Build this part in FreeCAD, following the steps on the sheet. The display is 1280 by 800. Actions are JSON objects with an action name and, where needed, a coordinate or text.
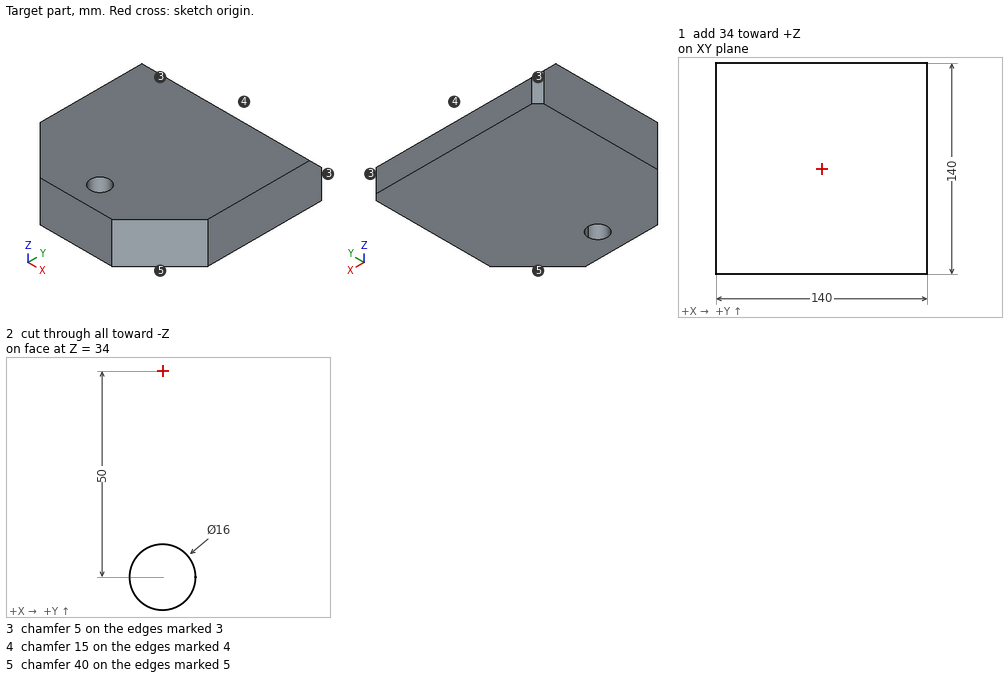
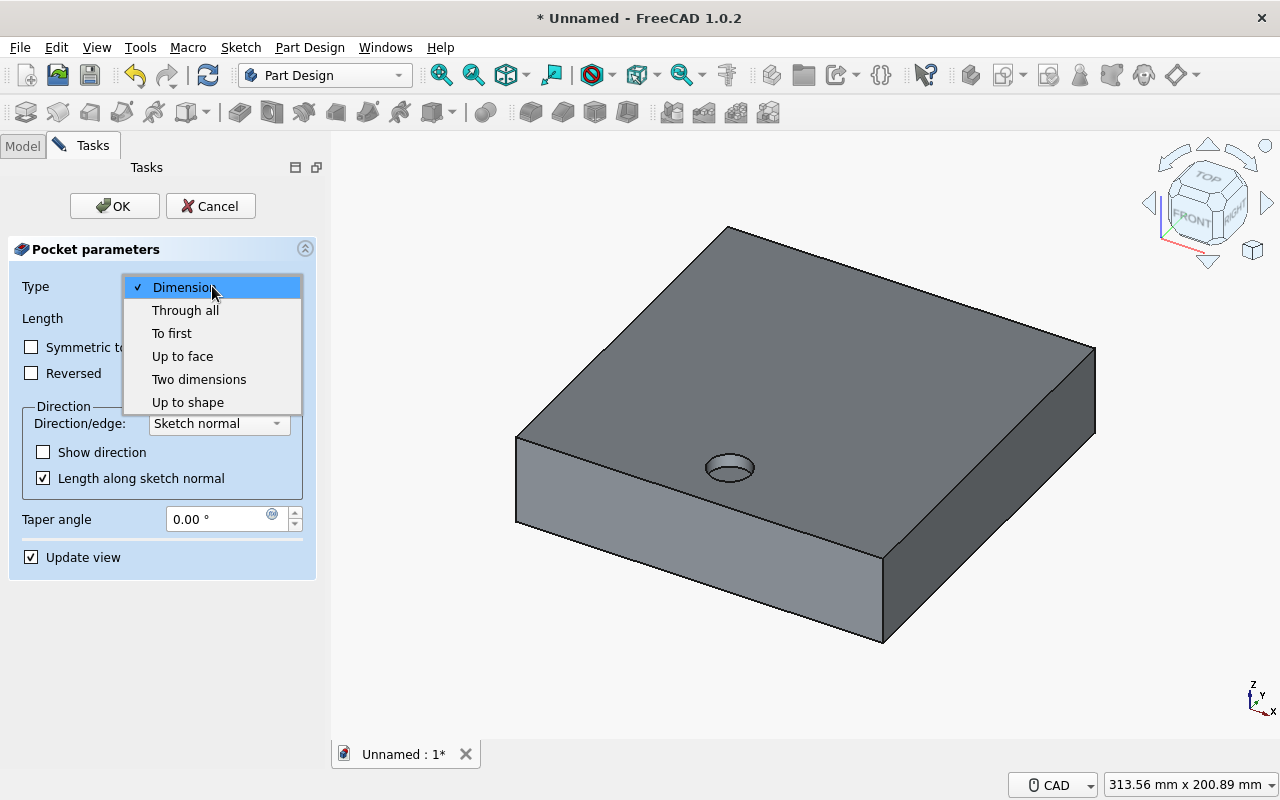
{"action": "left_click", "coordinate": [212, 310]}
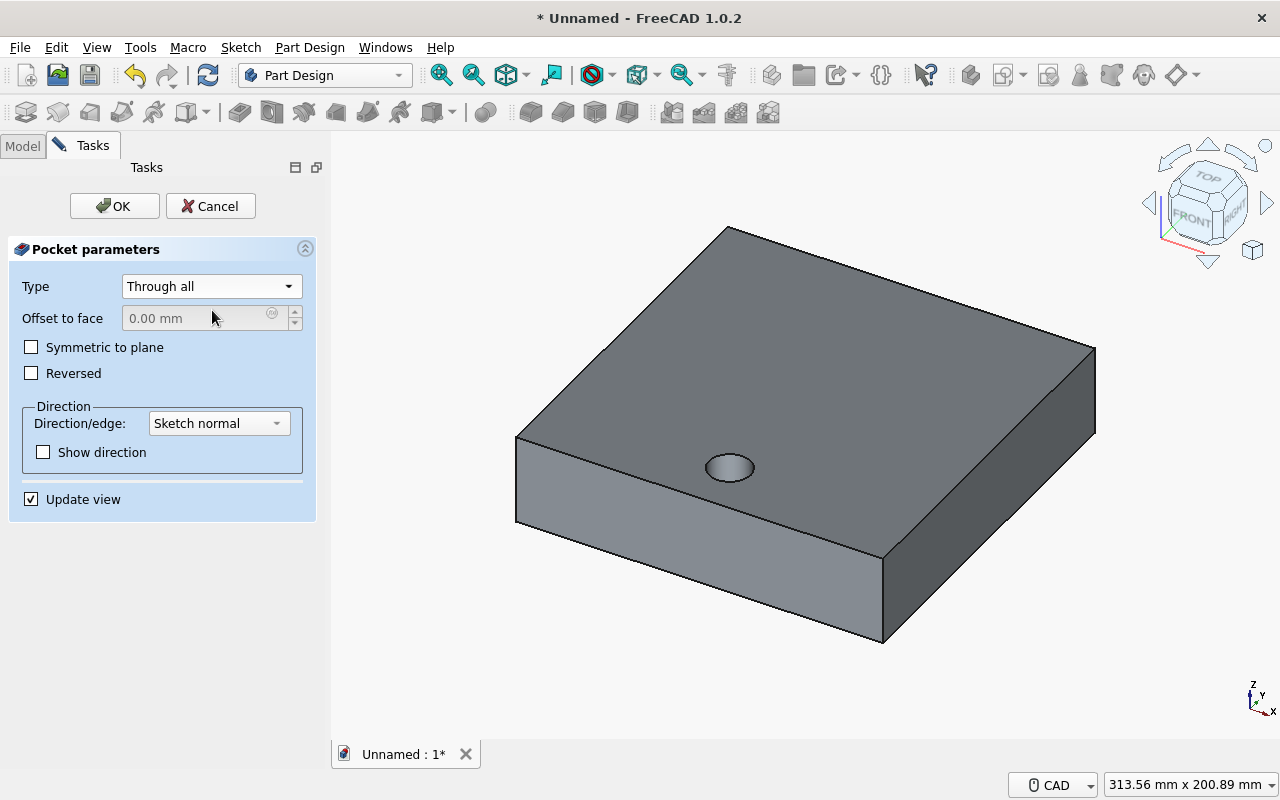
{"action": "left_click", "coordinate": [115, 206]}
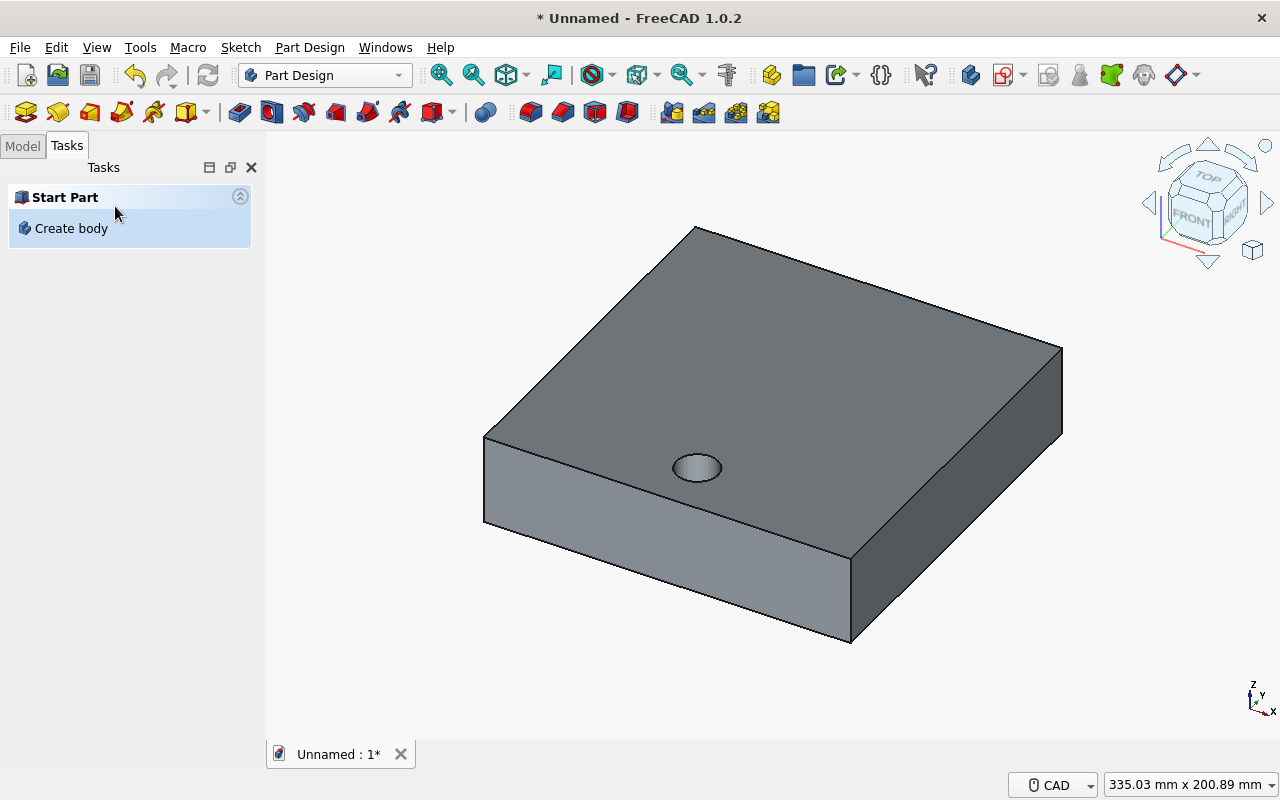
{"action": "key", "text": "0"}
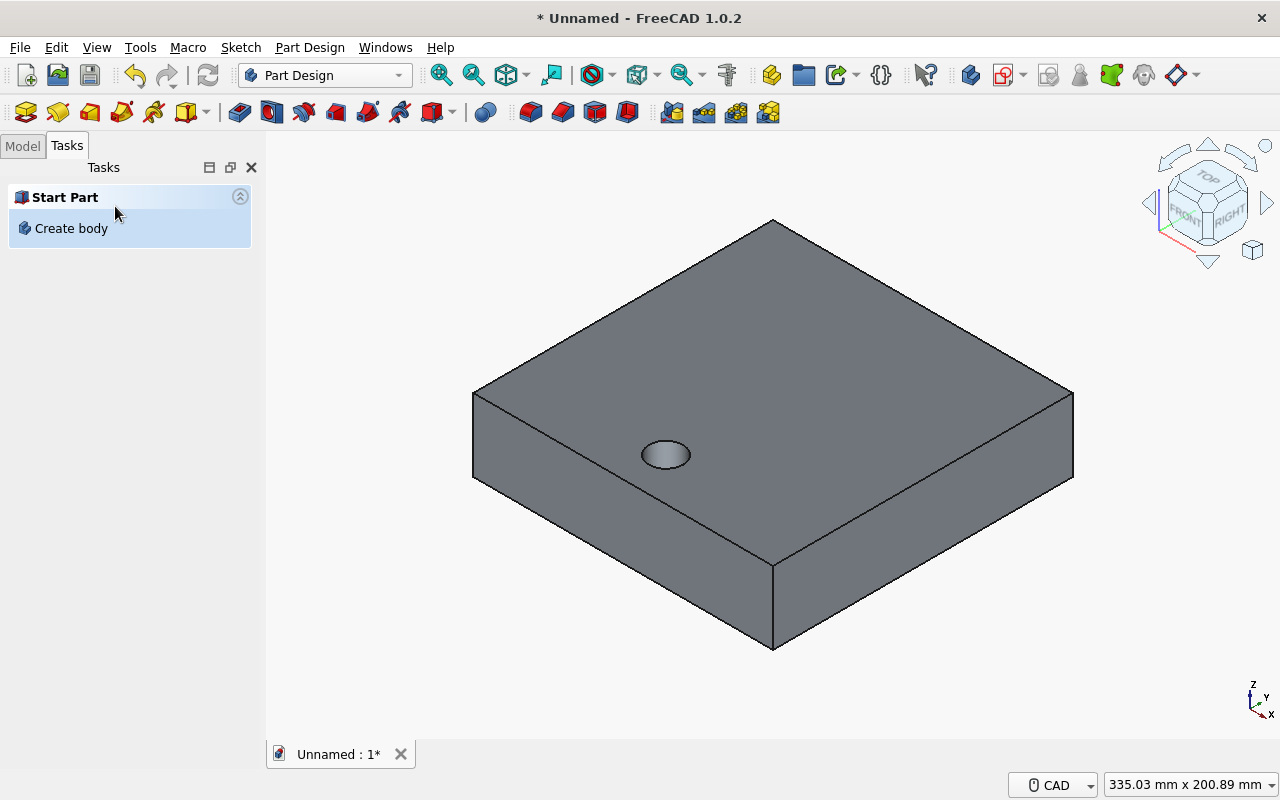
{"action": "key", "text": "2"}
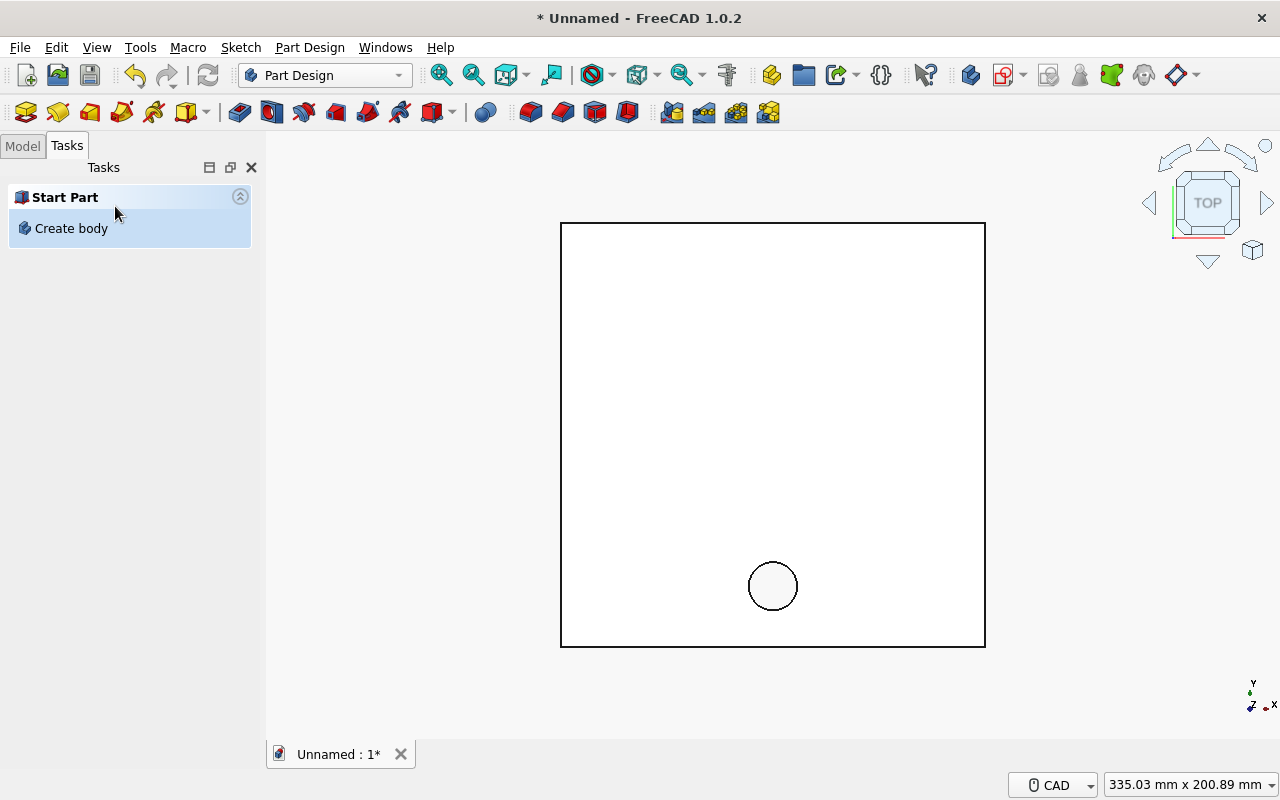
{"action": "key", "text": "1"}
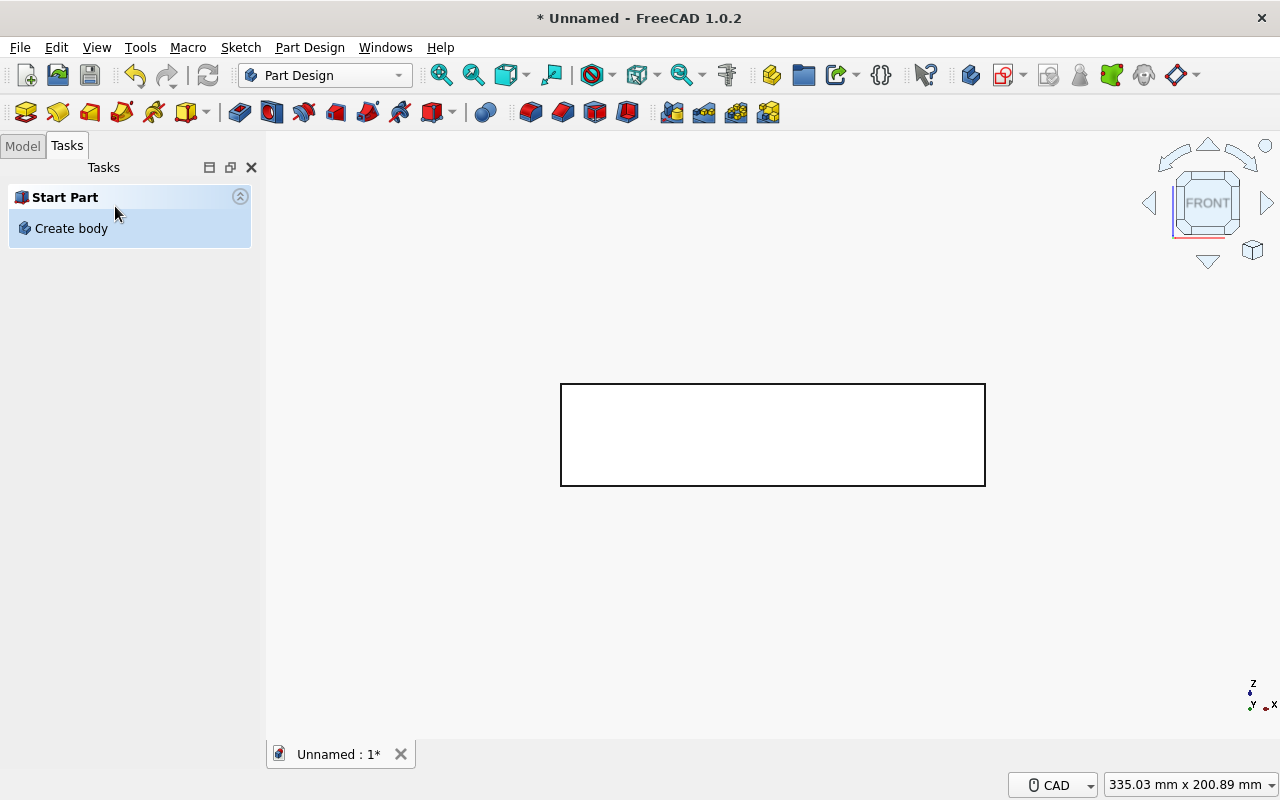
{"action": "key", "text": "v f"}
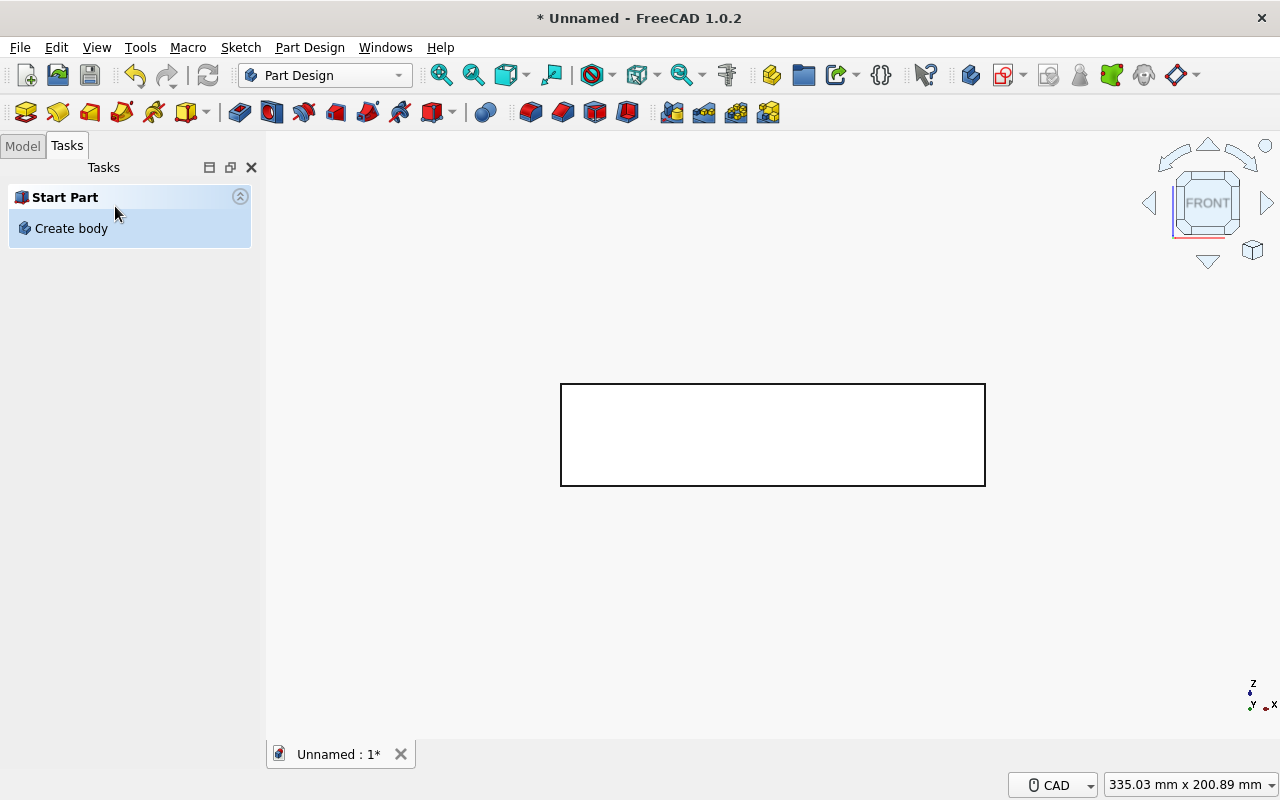
{"action": "key", "text": "3"}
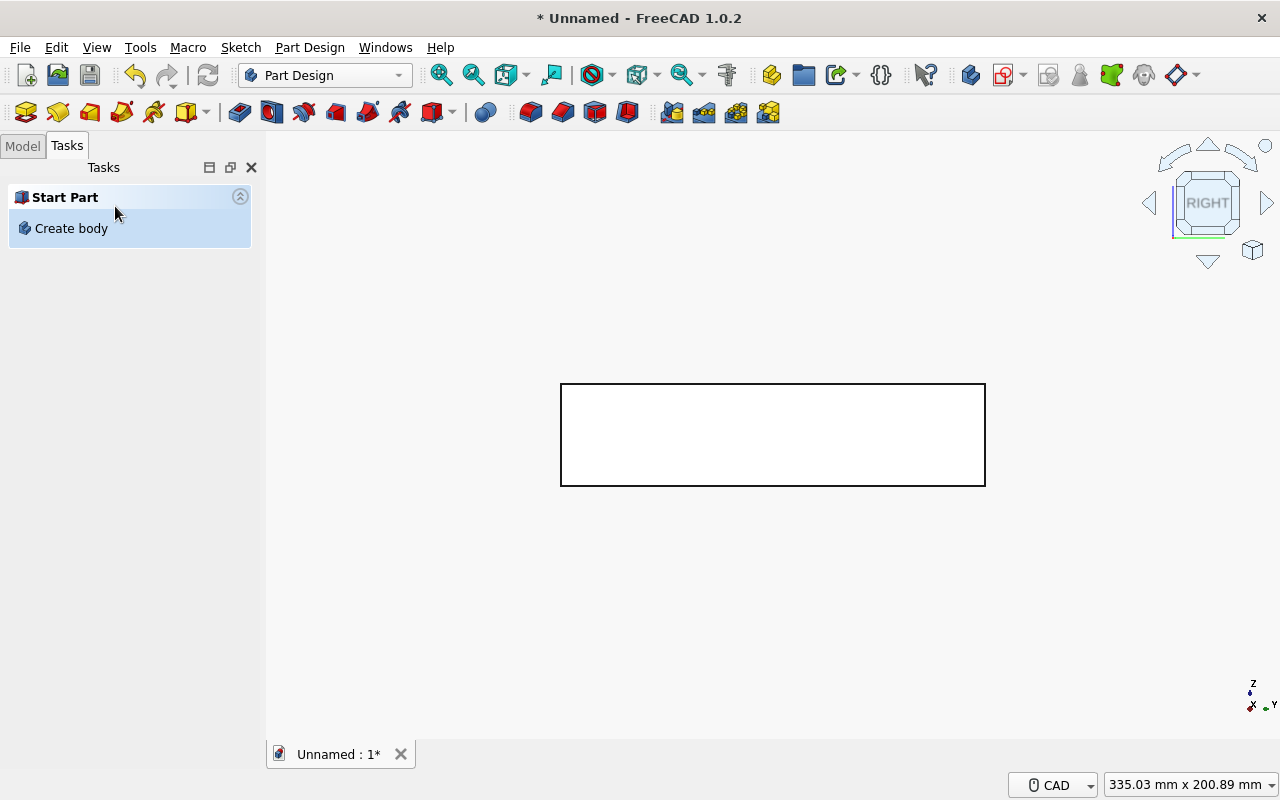
{"action": "key", "text": "v f"}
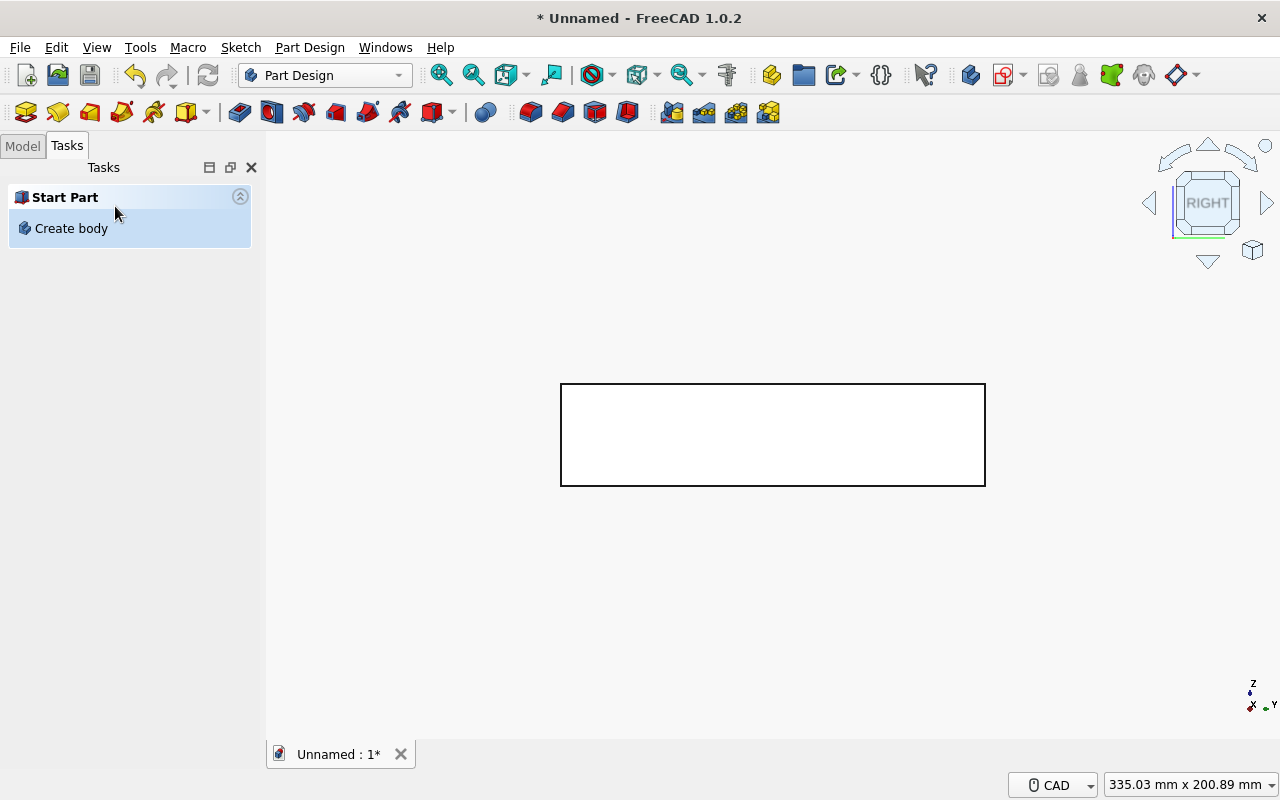
{"action": "left_click", "coordinate": [985, 434]}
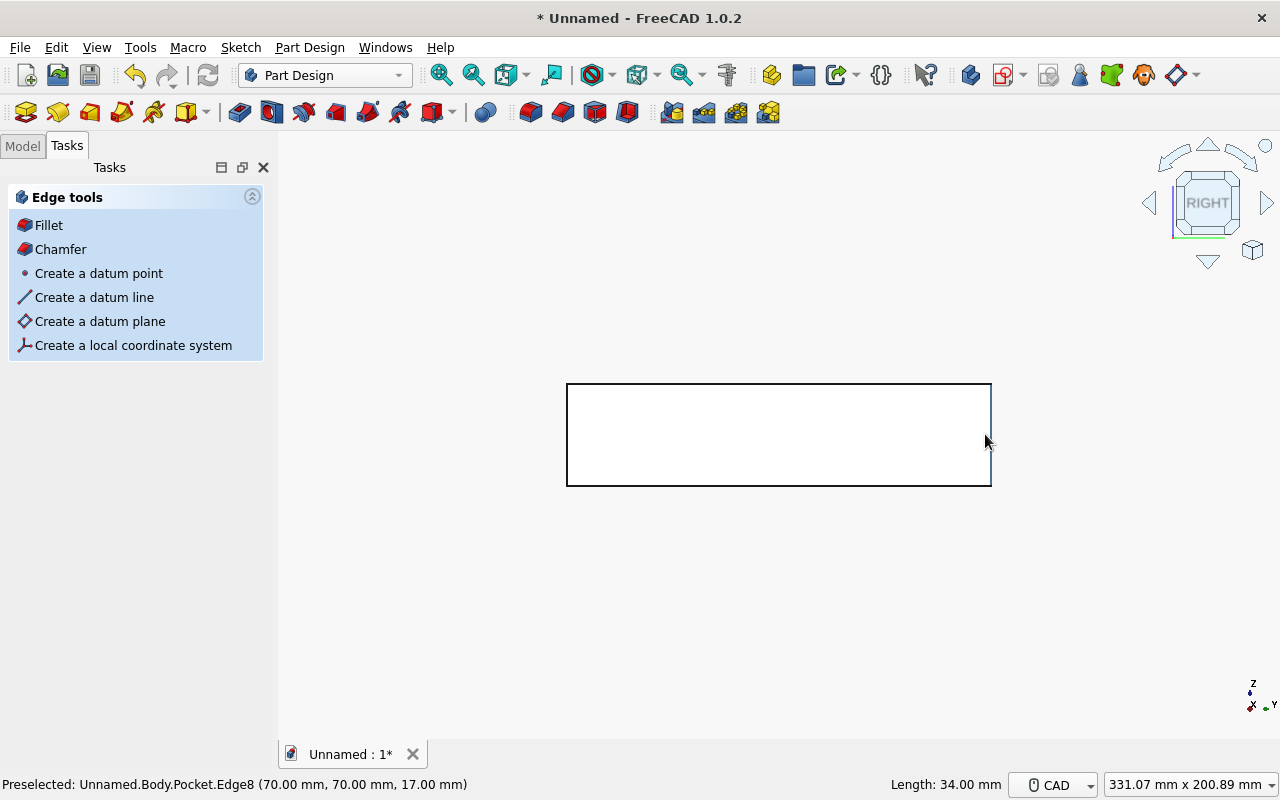
{"action": "key", "text": "5"}